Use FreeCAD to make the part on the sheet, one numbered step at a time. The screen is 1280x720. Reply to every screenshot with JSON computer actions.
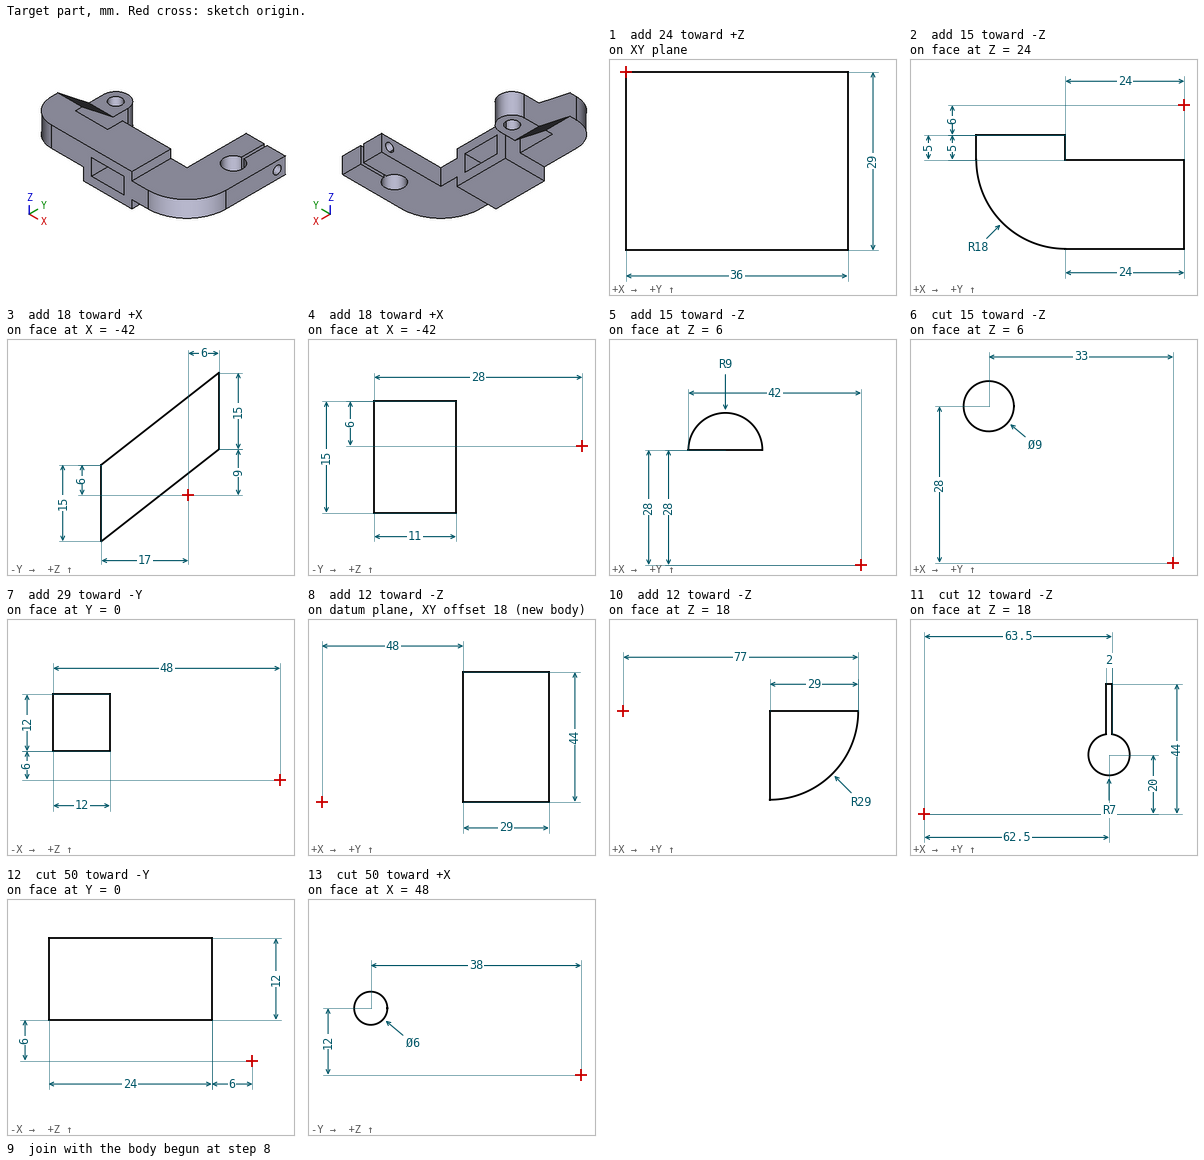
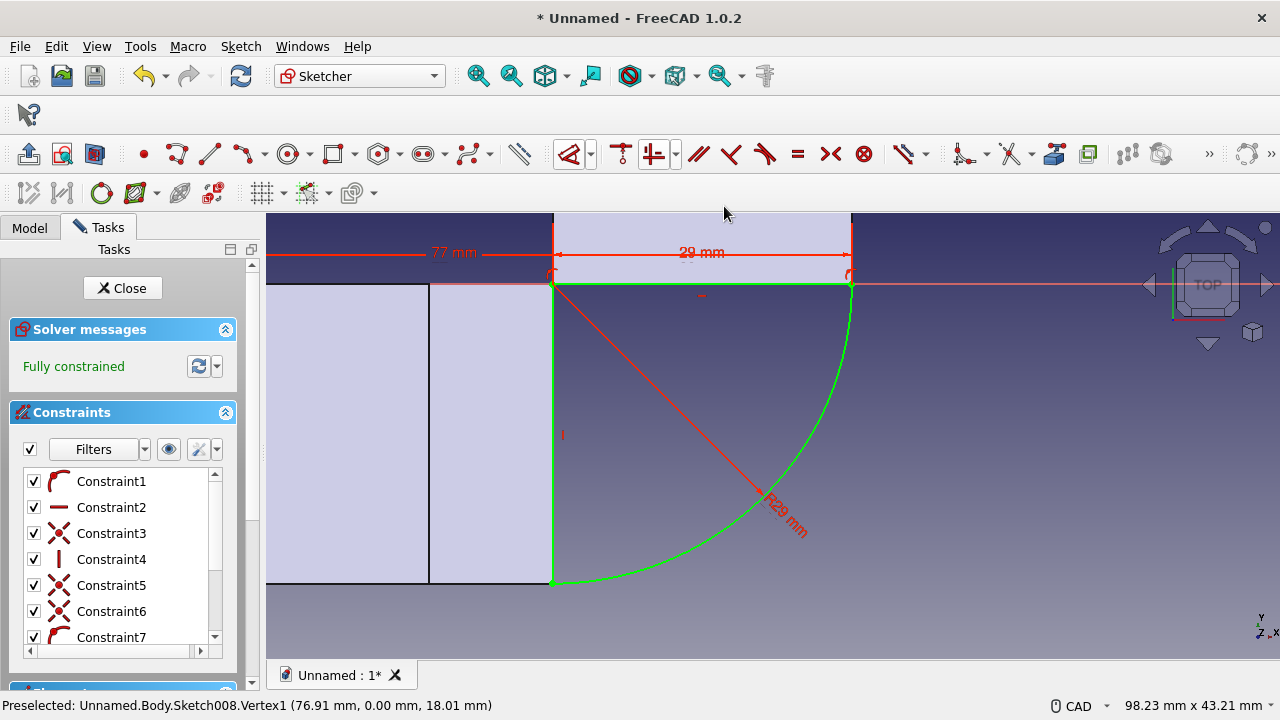
{"action": "left_click", "coordinate": [123, 288]}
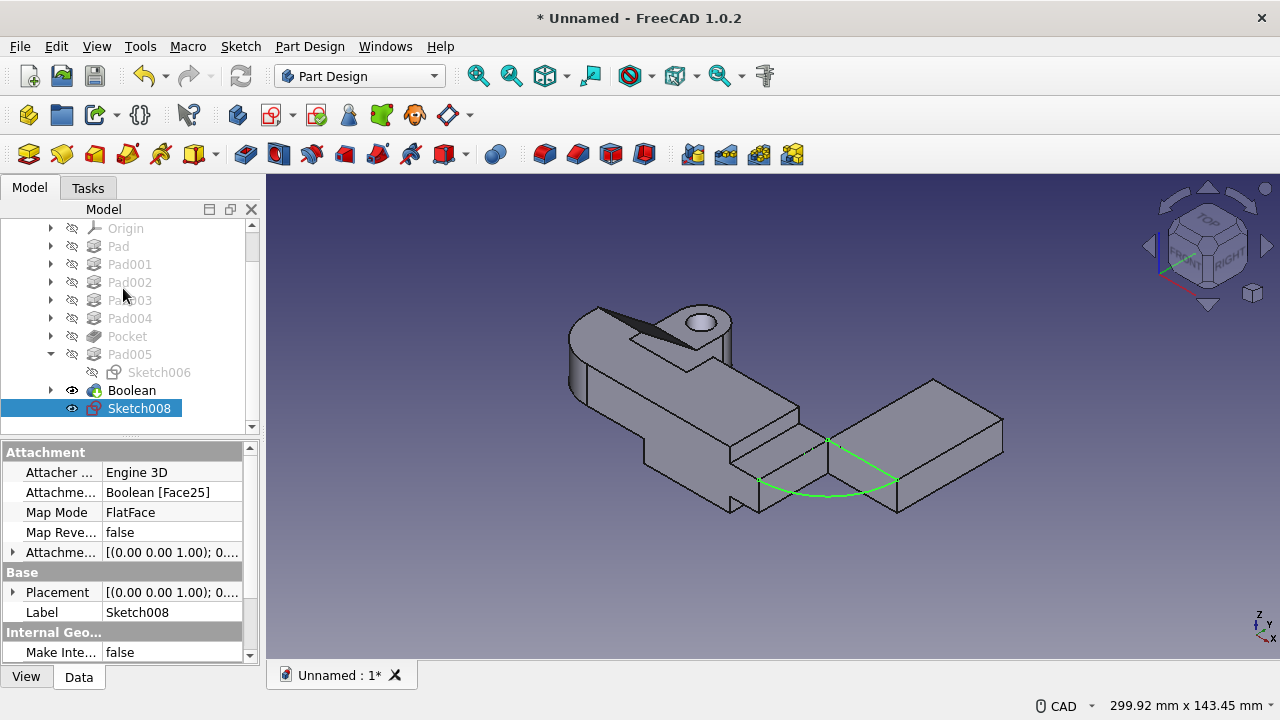
{"action": "left_click", "coordinate": [29, 154]}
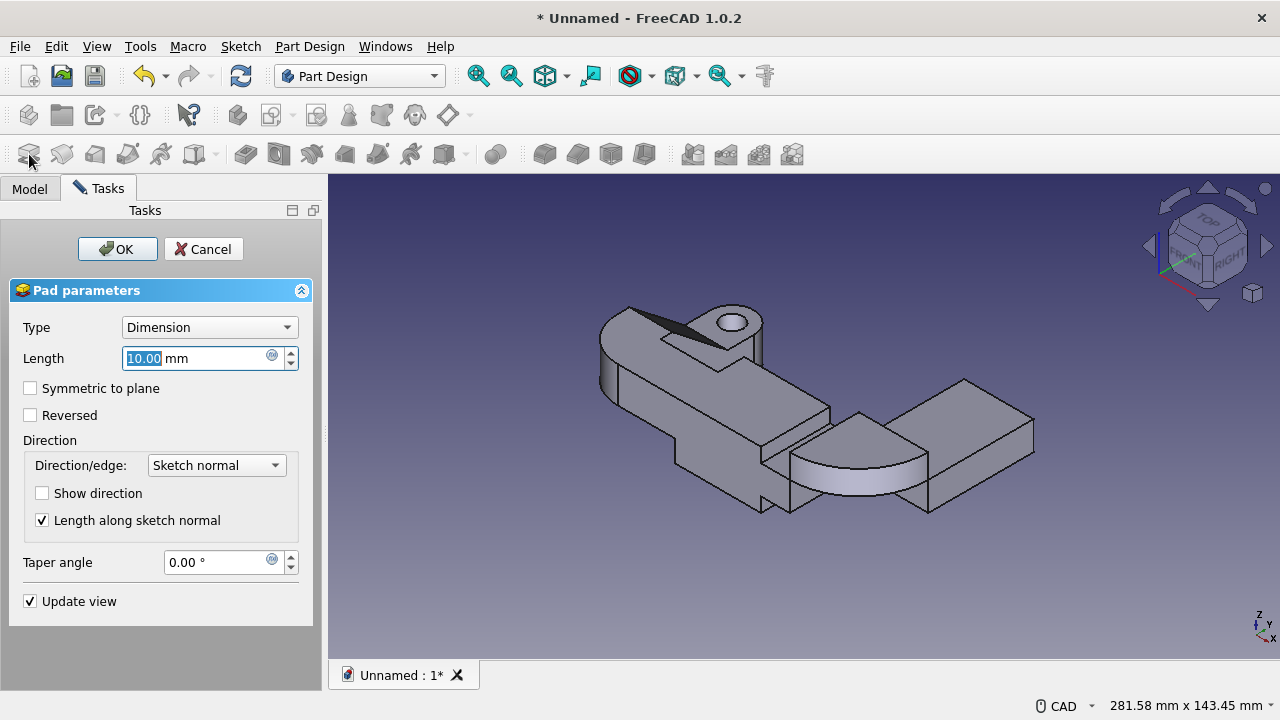
{"action": "type", "text": "12"}
{"action": "key", "text": "Tab"}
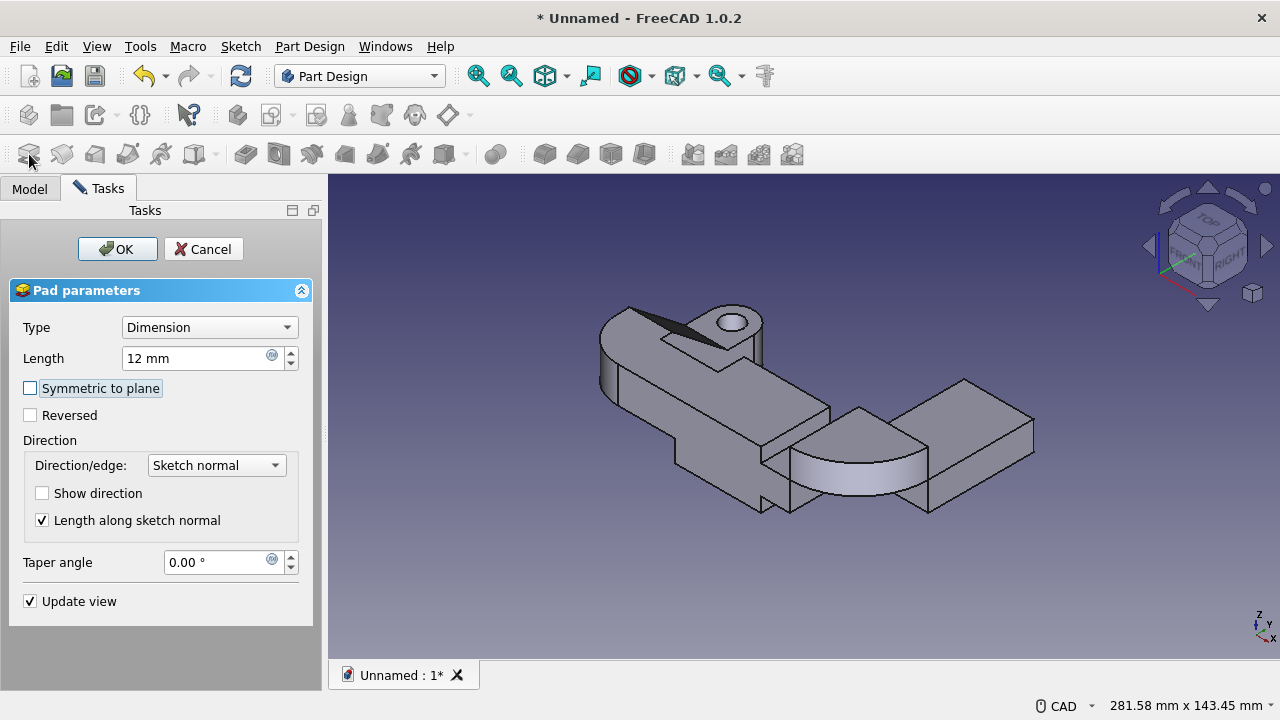
{"action": "left_click", "coordinate": [31, 415]}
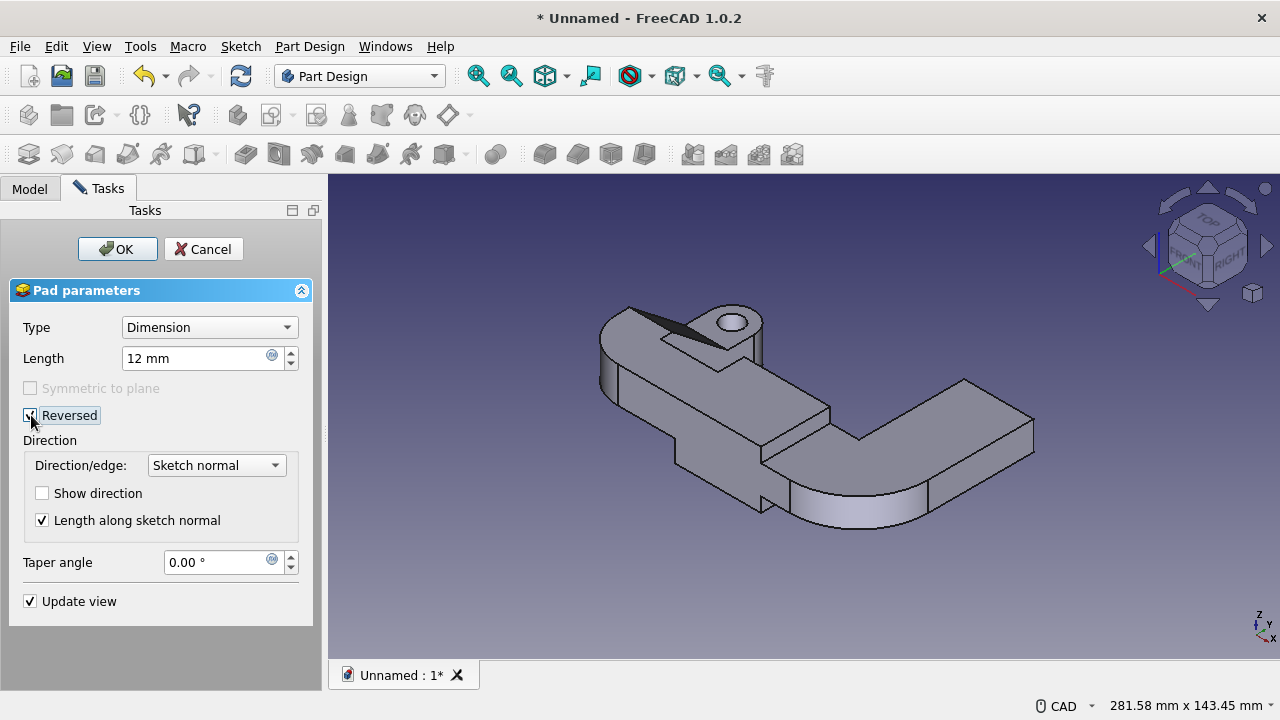
{"action": "left_click", "coordinate": [118, 249]}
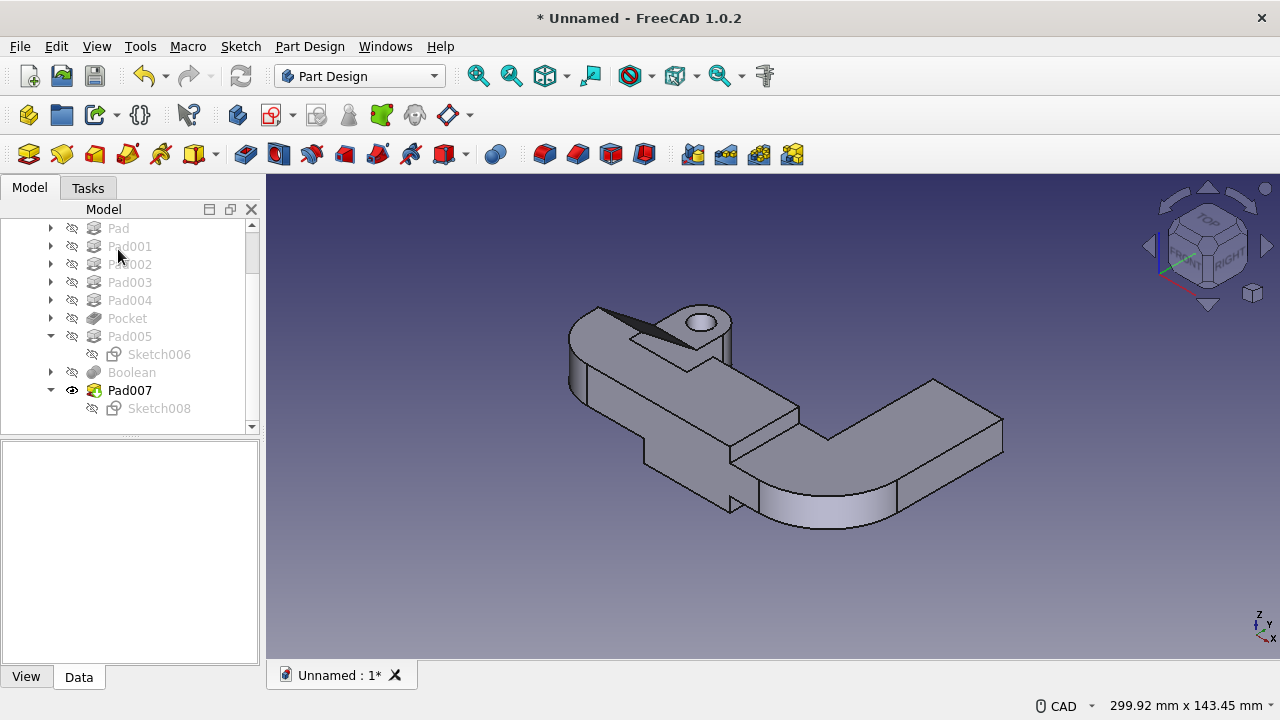
{"action": "left_click", "coordinate": [930, 420]}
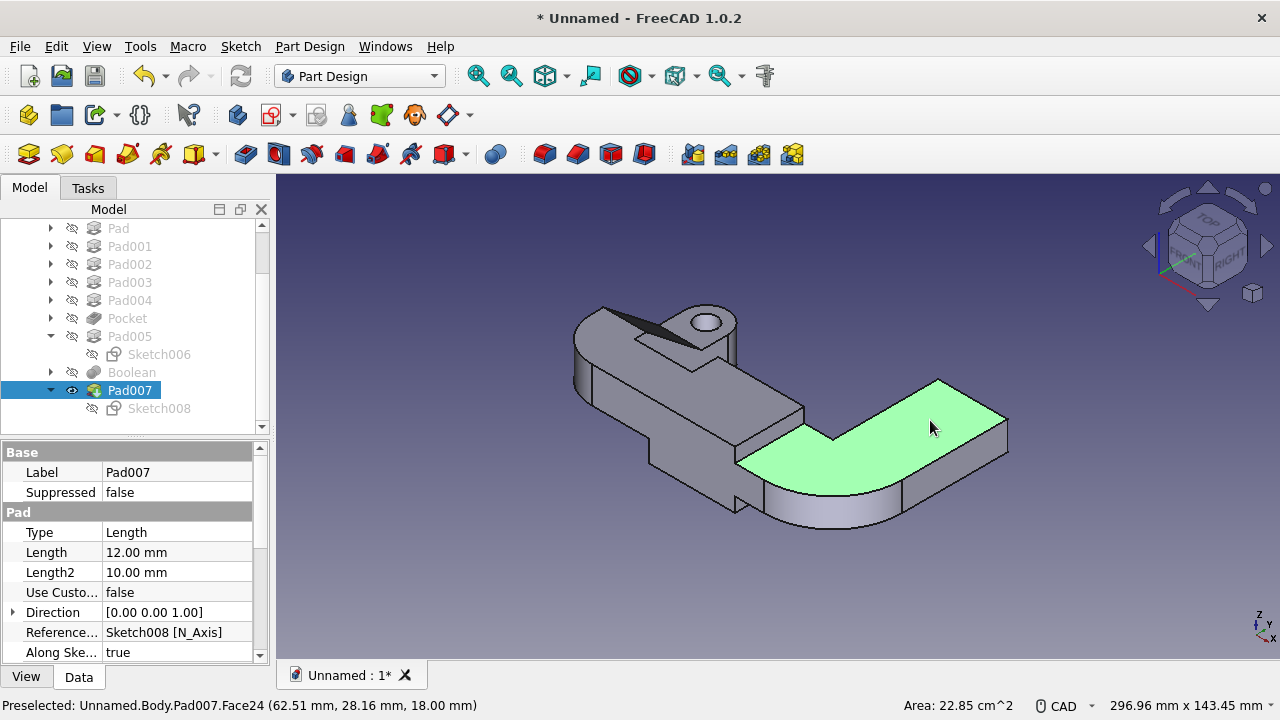
{"action": "left_click", "coordinate": [270, 116]}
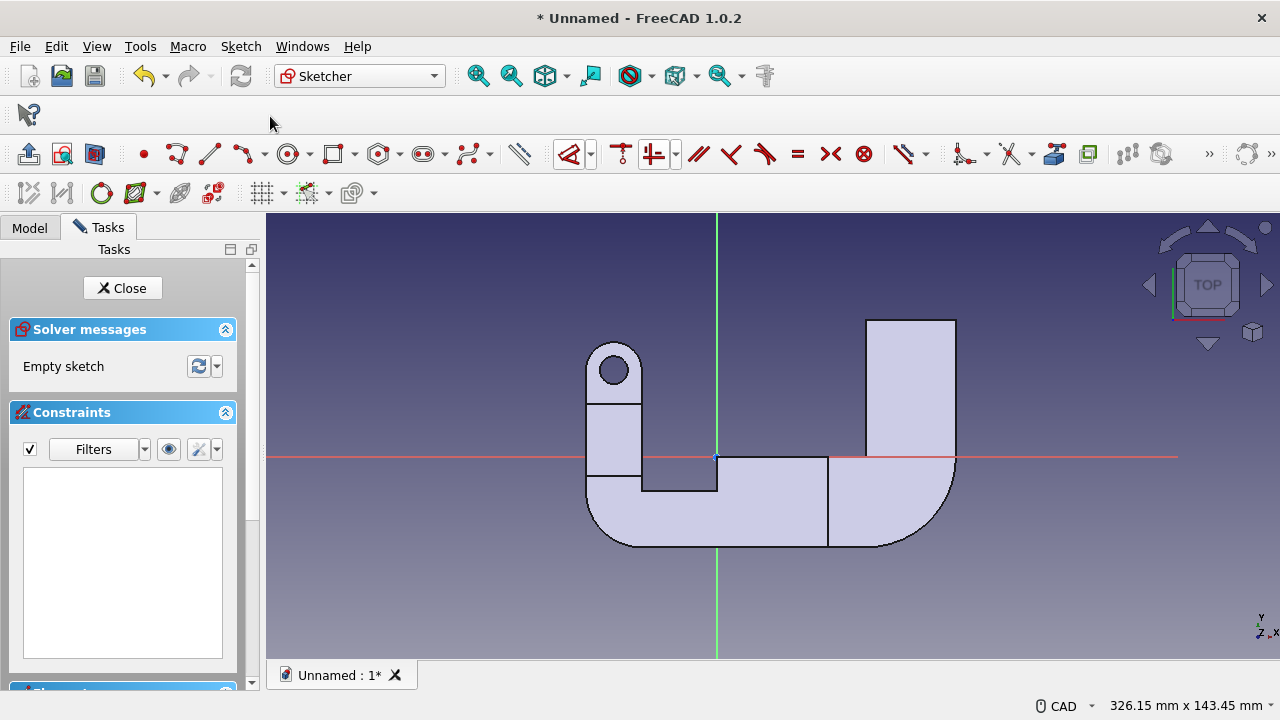
{"action": "scroll", "coordinate": [950, 331], "scroll_direction": "up", "scroll_amount": 3}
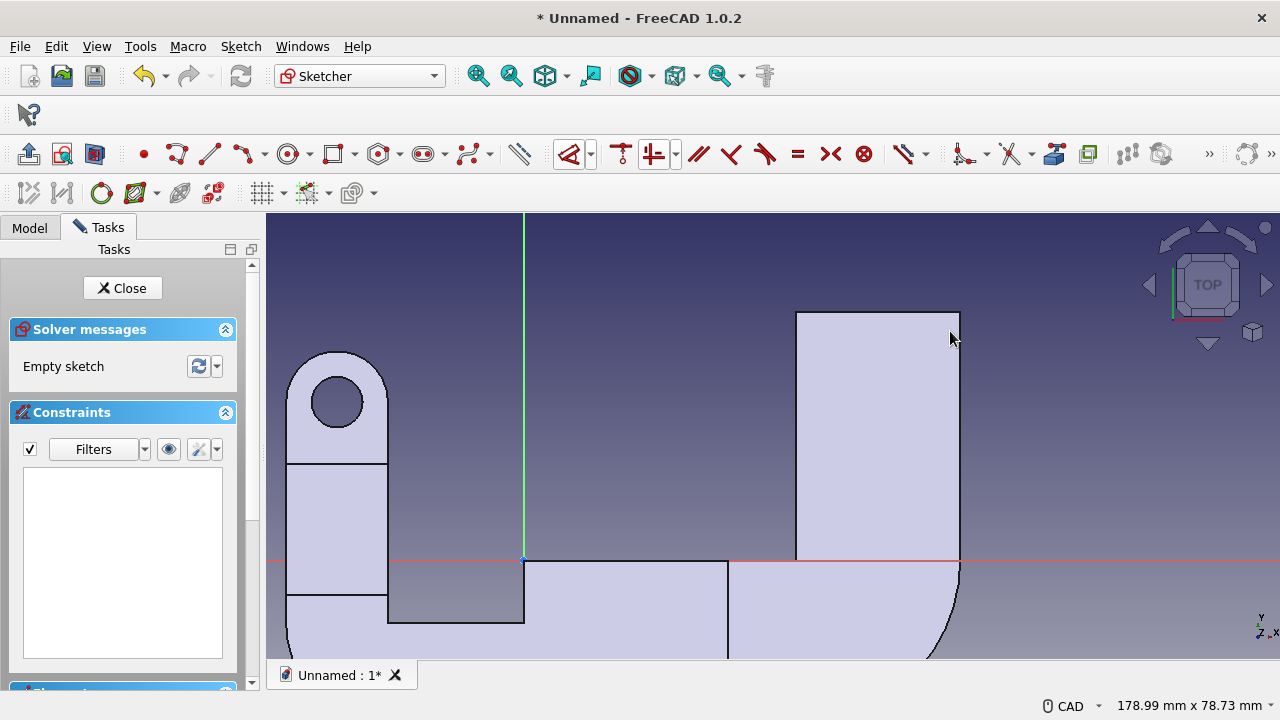
{"action": "key", "text": "g m"}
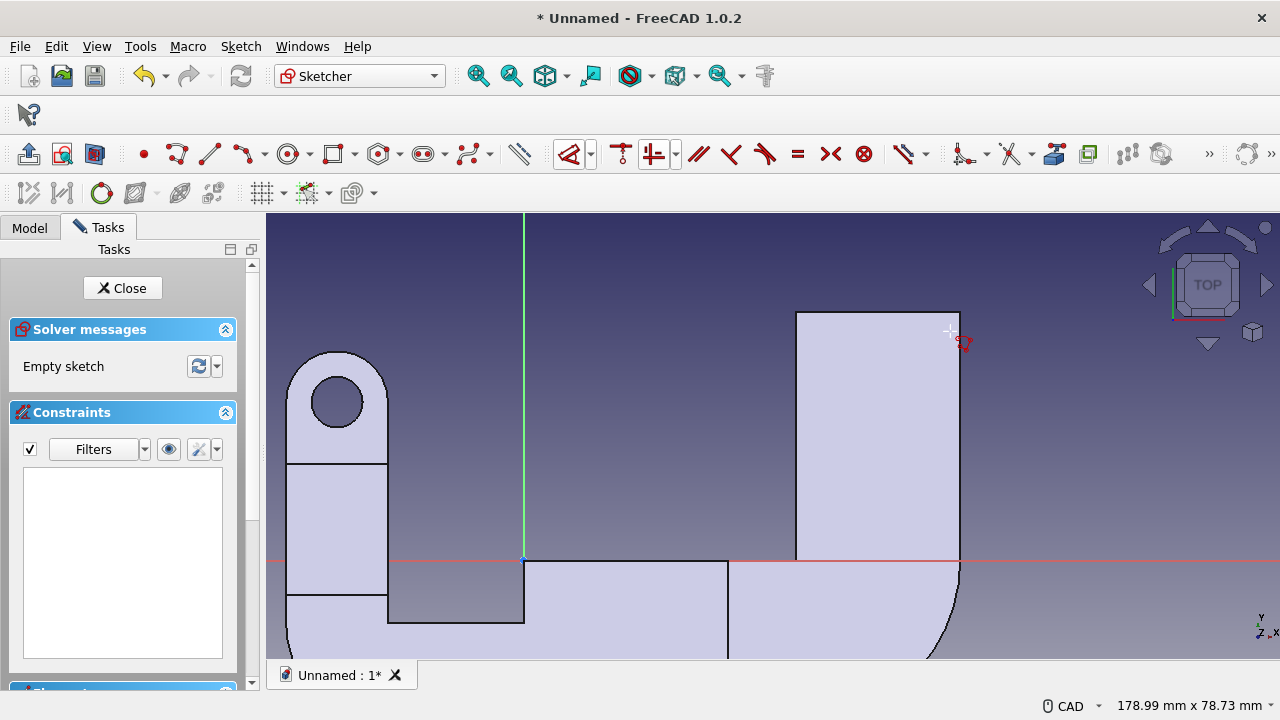
{"action": "left_click", "coordinate": [884, 408]}
{"action": "left_click", "coordinate": [884, 312]}